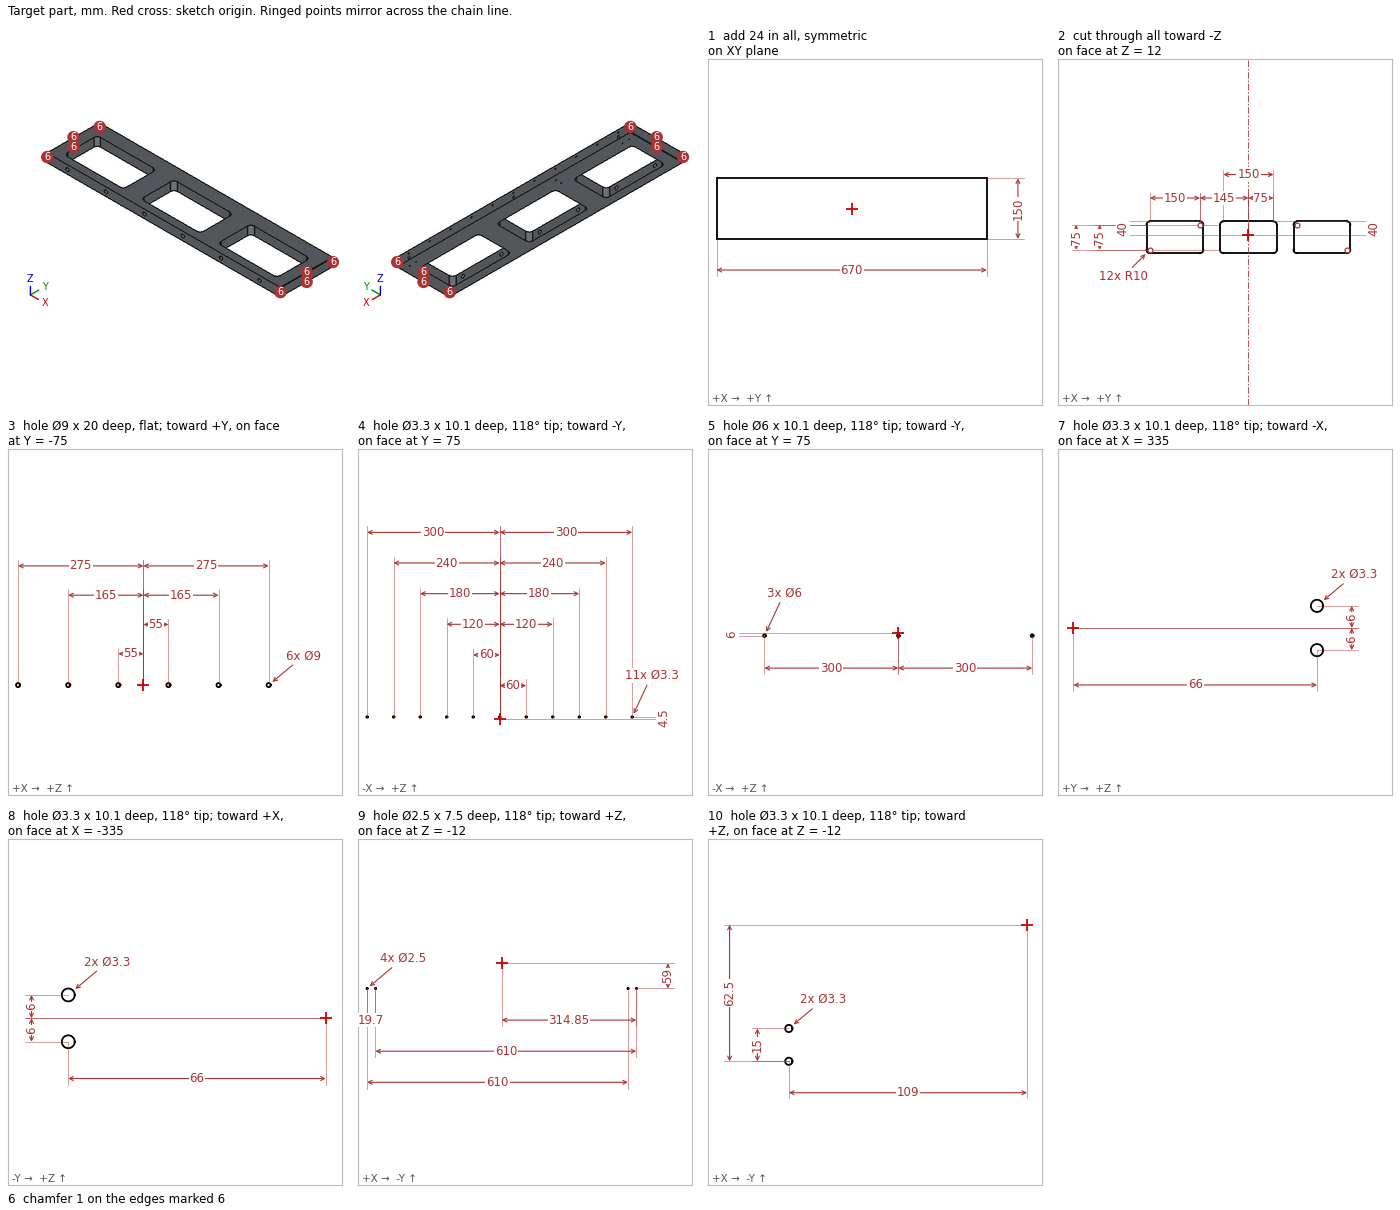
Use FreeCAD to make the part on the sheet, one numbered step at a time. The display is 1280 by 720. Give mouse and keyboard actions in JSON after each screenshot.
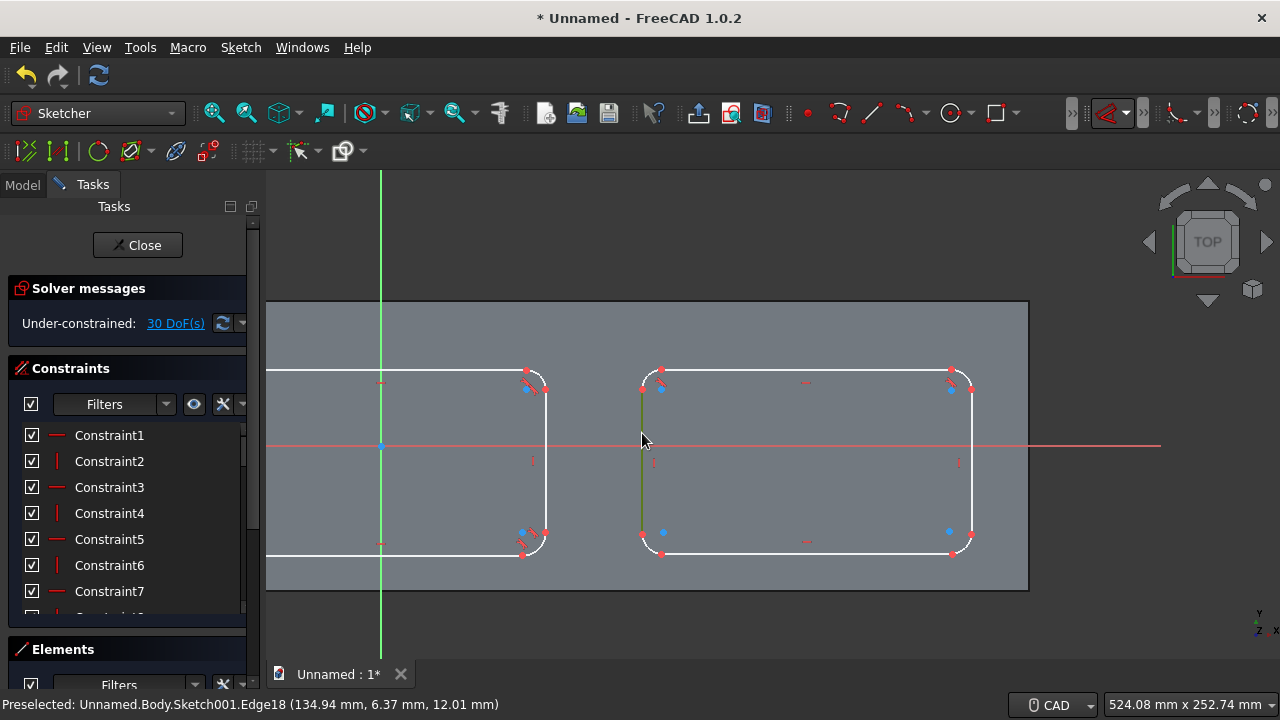
{"action": "scroll", "coordinate": [653, 372], "scroll_direction": "up", "scroll_amount": 2}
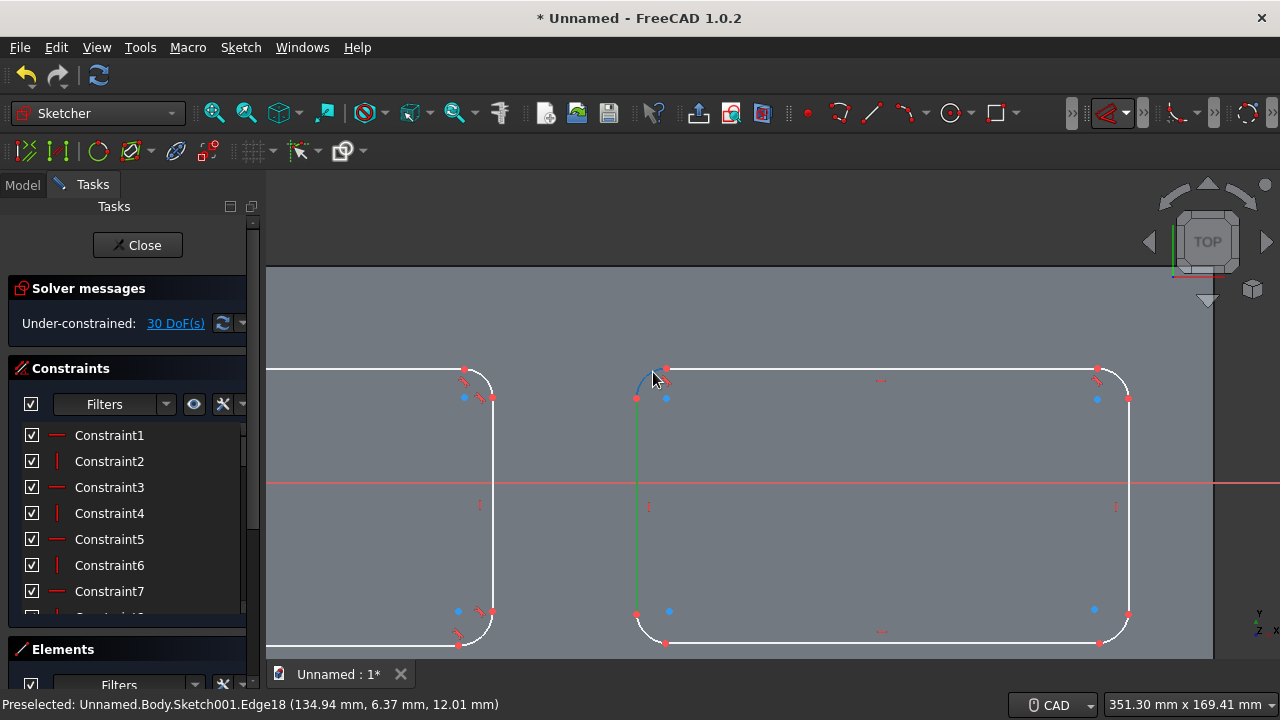
{"action": "left_click", "coordinate": [653, 372]}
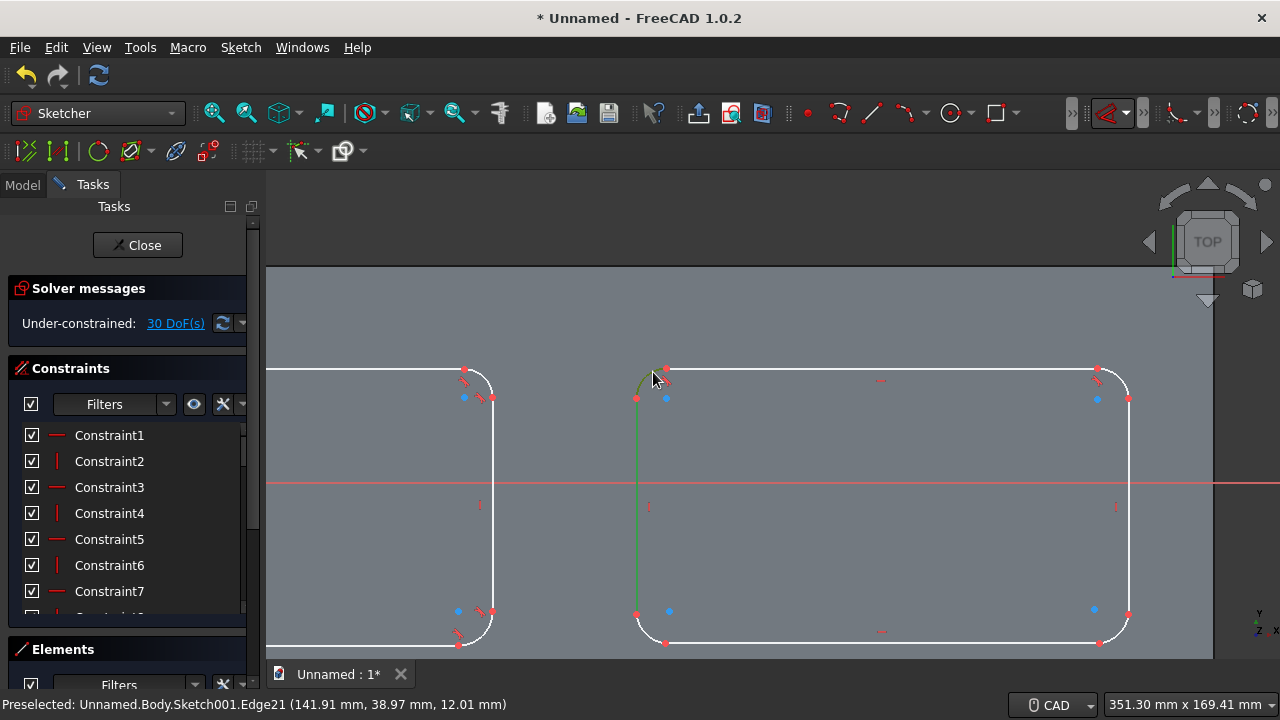
{"action": "key", "text": "t"}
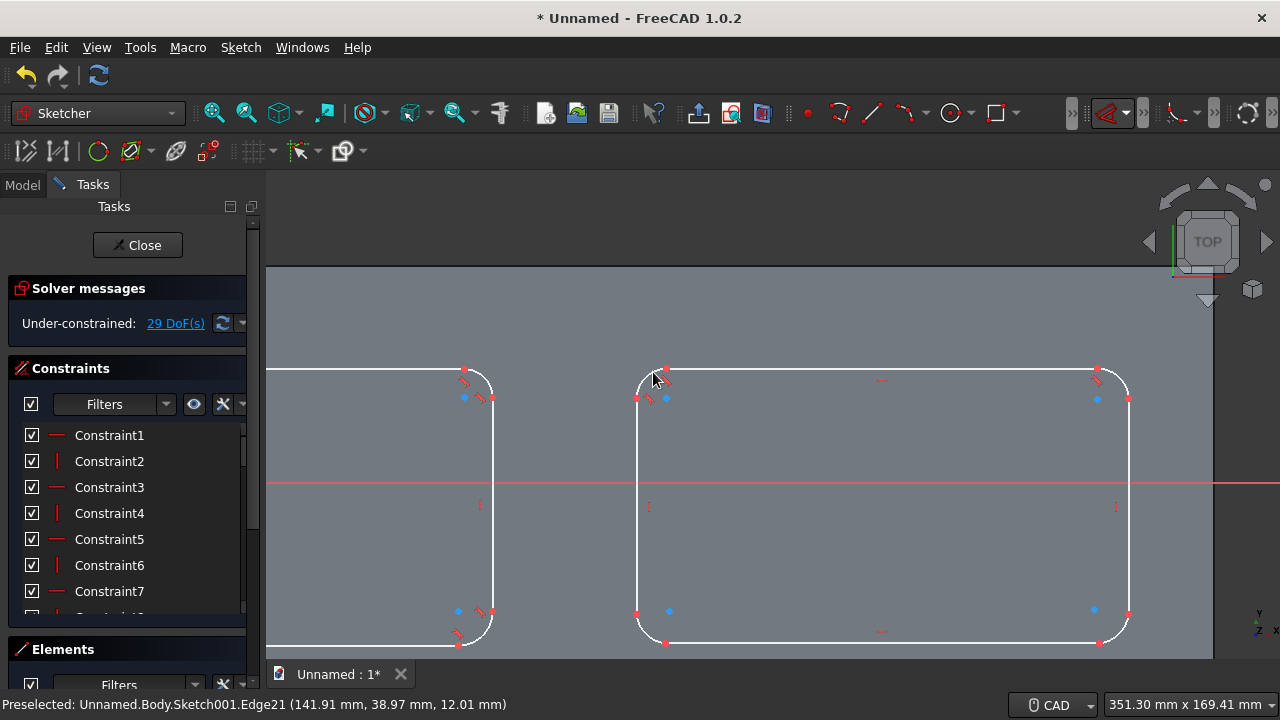
{"action": "left_click", "coordinate": [637, 463]}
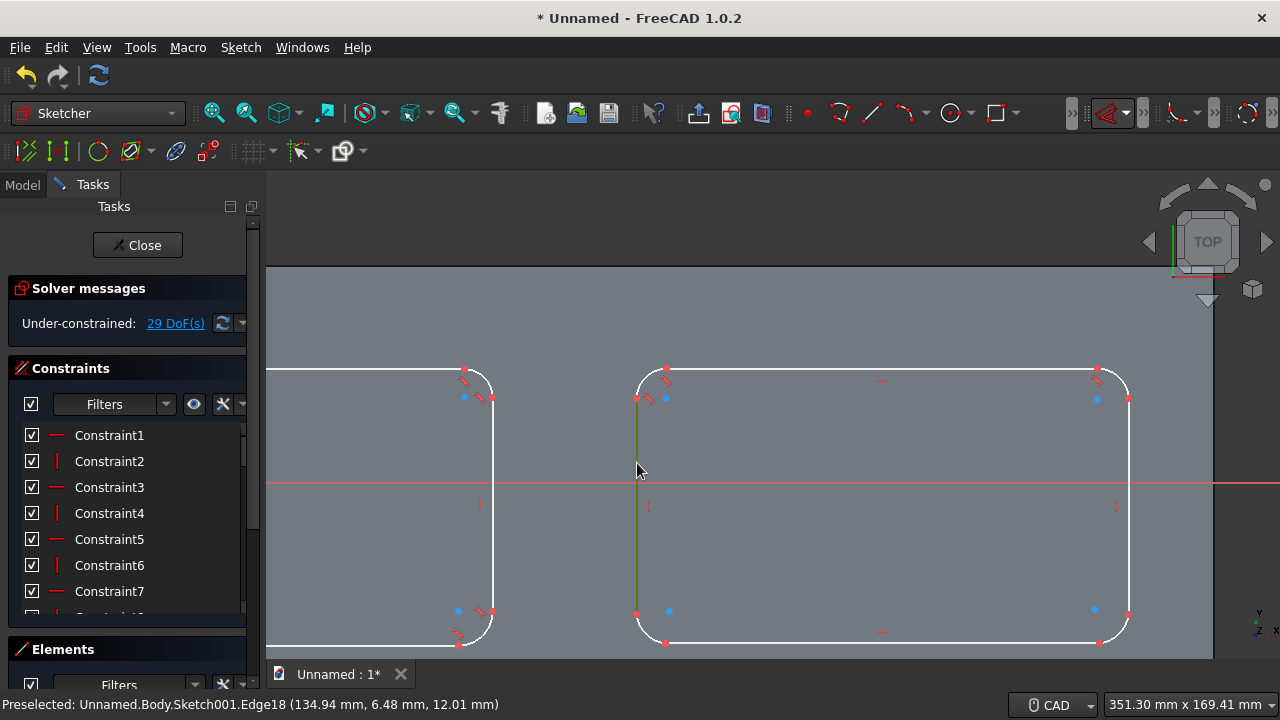
{"action": "left_click", "coordinate": [641, 627]}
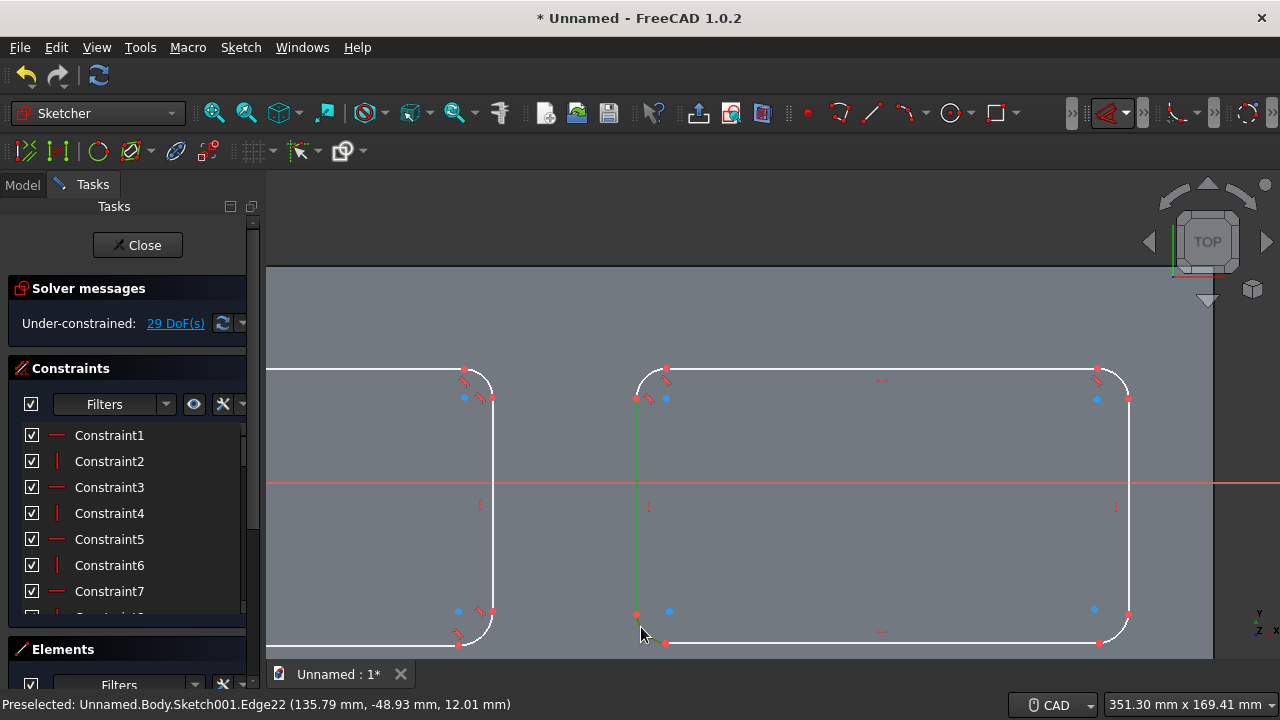
{"action": "key", "text": "t"}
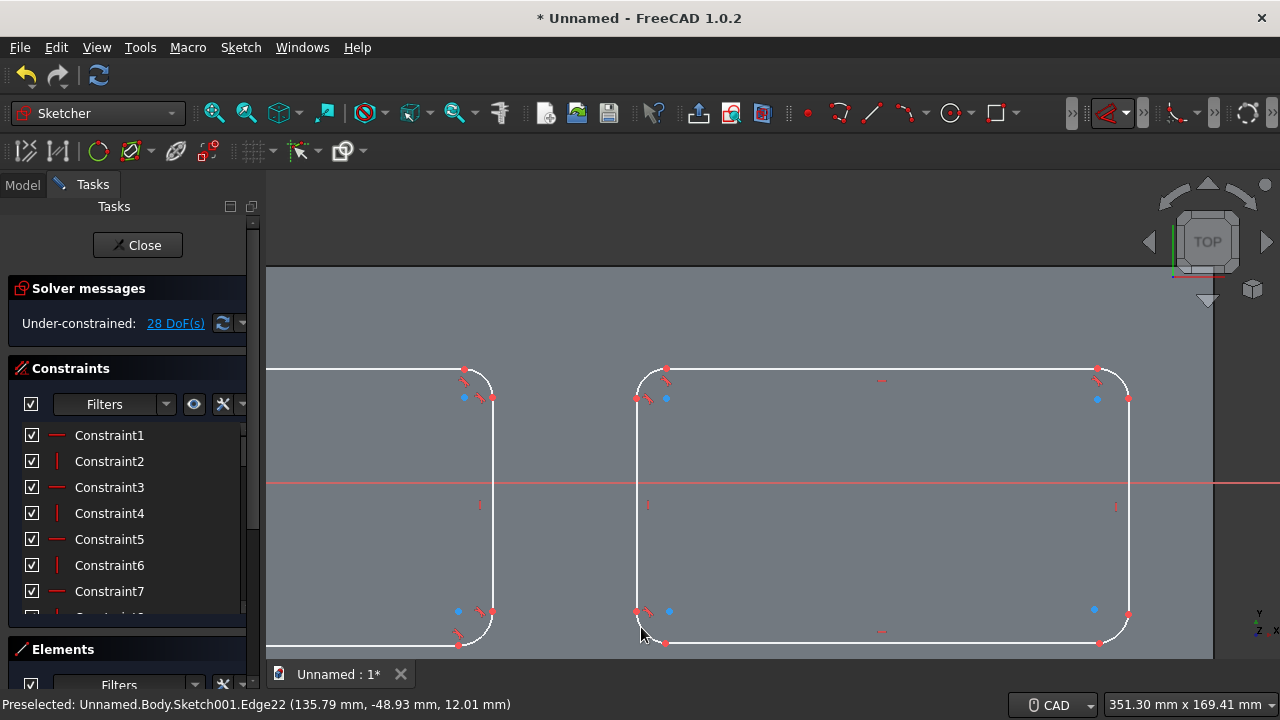
{"action": "scroll", "coordinate": [902, 376], "scroll_direction": "down", "scroll_amount": 6}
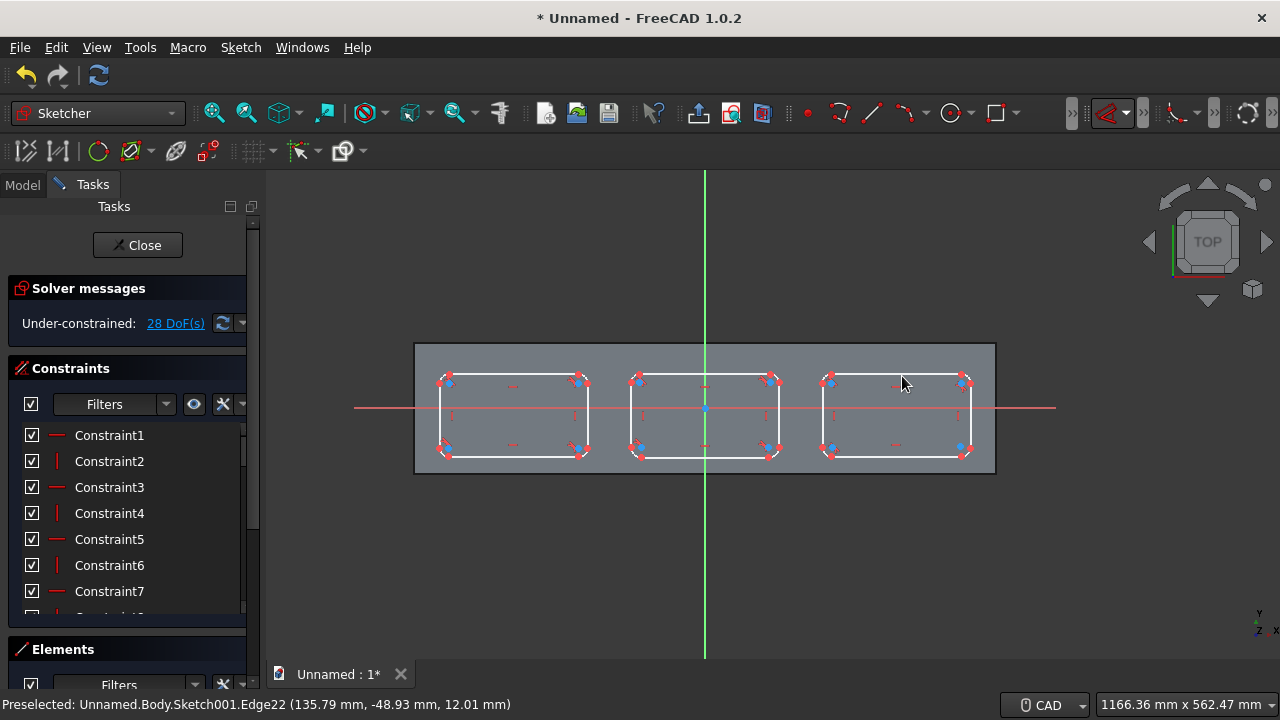
{"action": "left_click", "coordinate": [870, 457]}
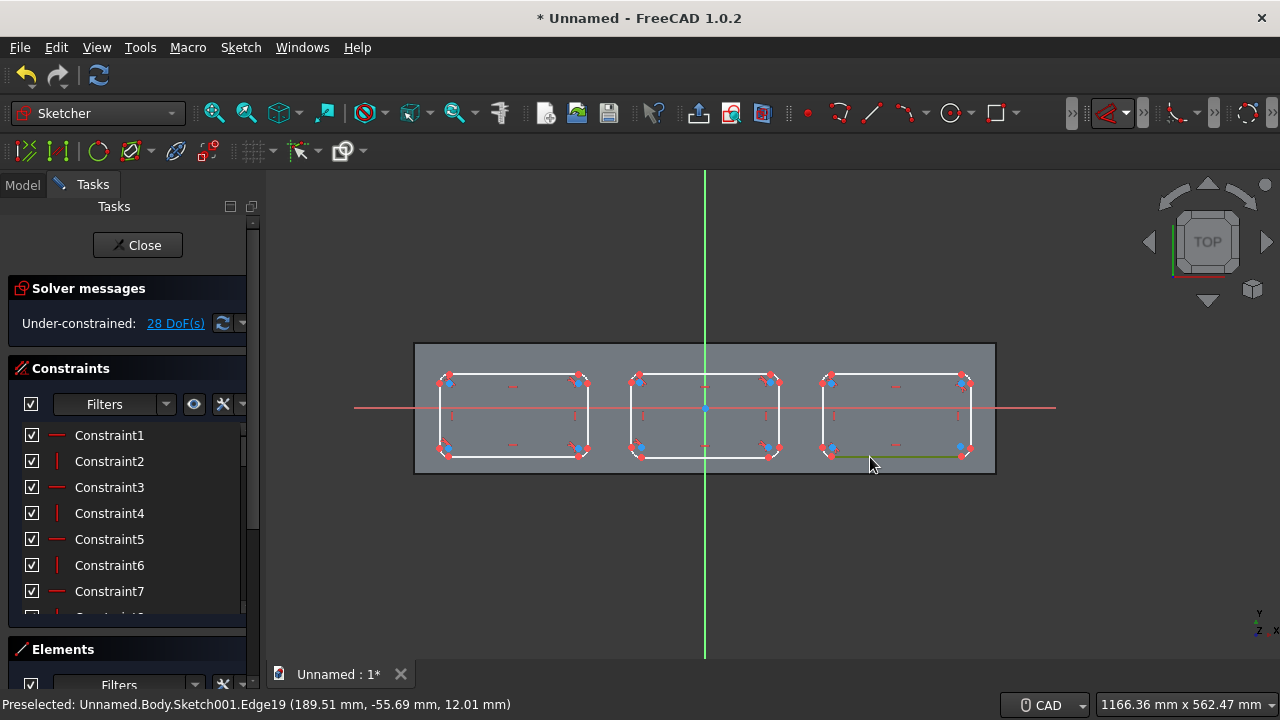
{"action": "scroll", "coordinate": [825, 454], "scroll_direction": "up", "scroll_amount": 4}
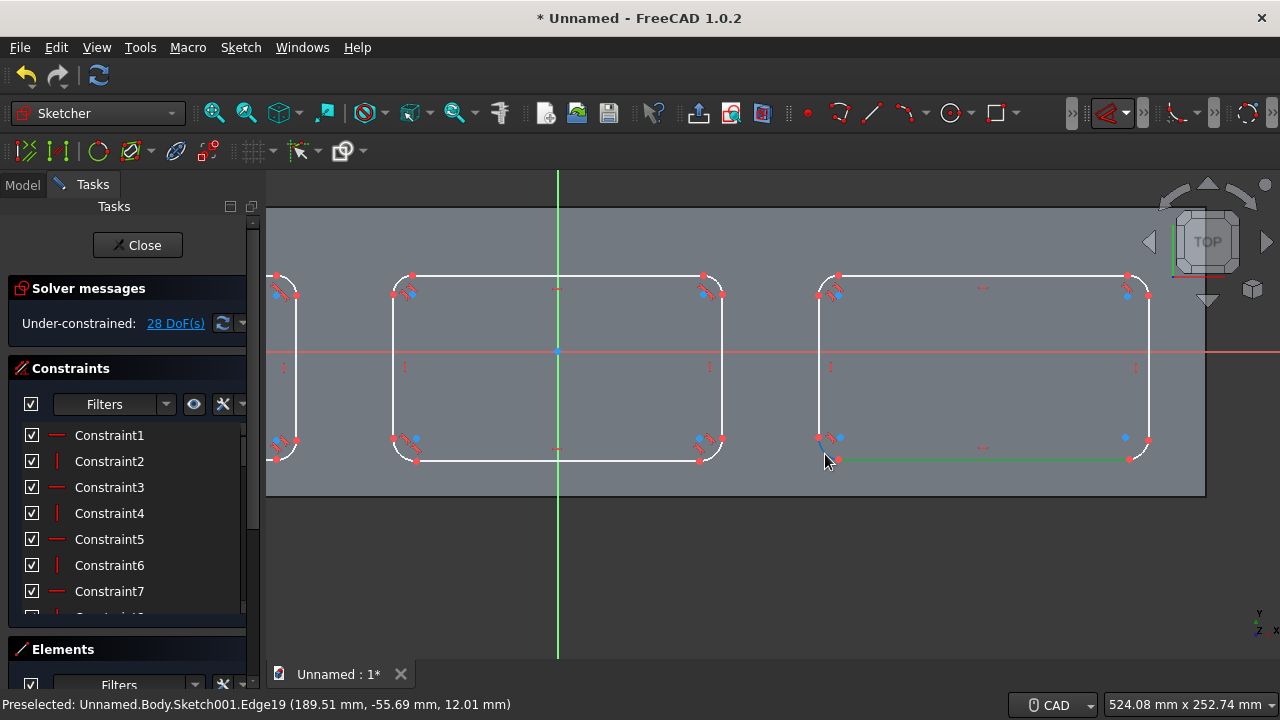
{"action": "left_click", "coordinate": [824, 453]}